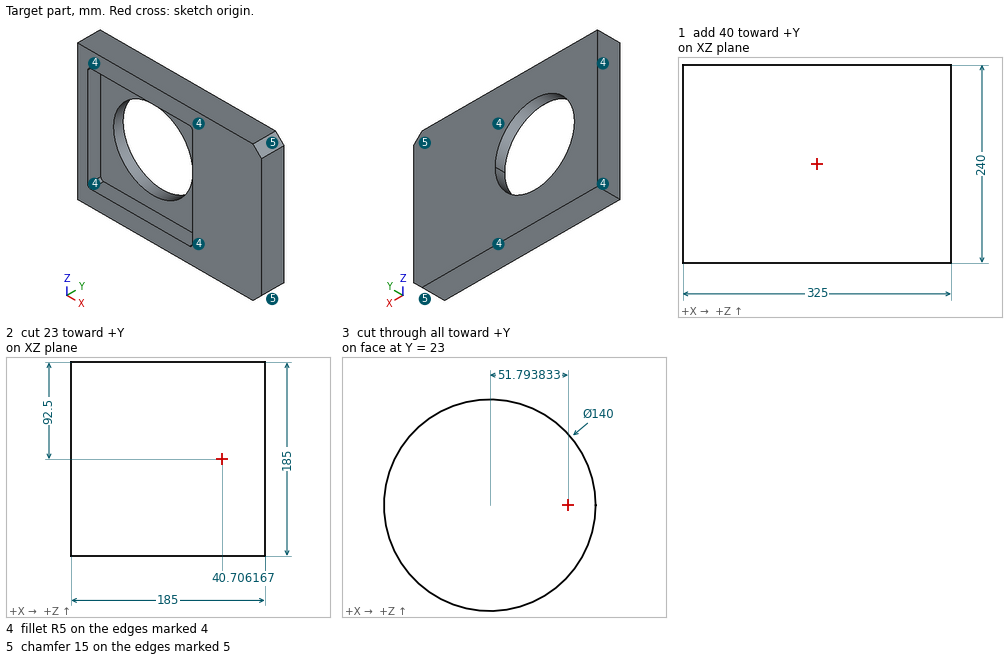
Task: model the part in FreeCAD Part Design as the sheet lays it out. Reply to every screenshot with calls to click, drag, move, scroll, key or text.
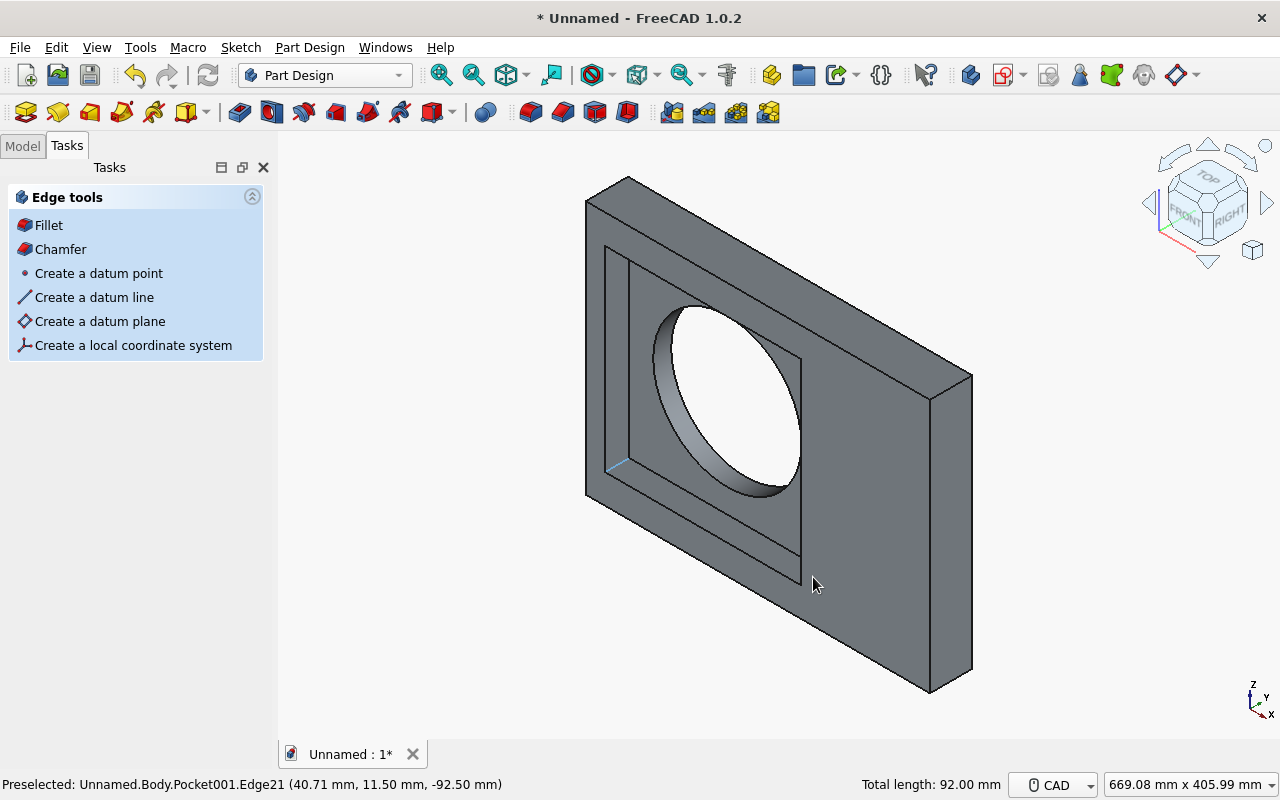
click(532, 112)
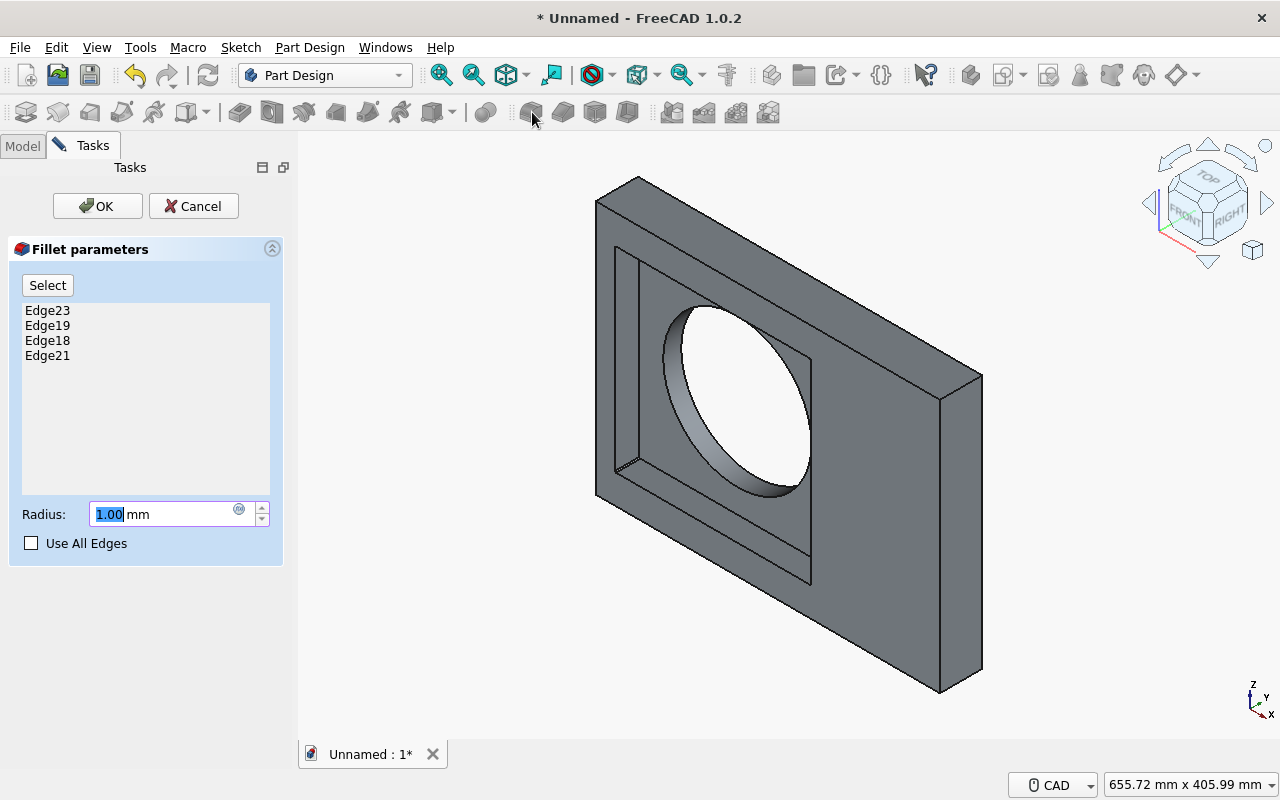
text(5)
key(Tab)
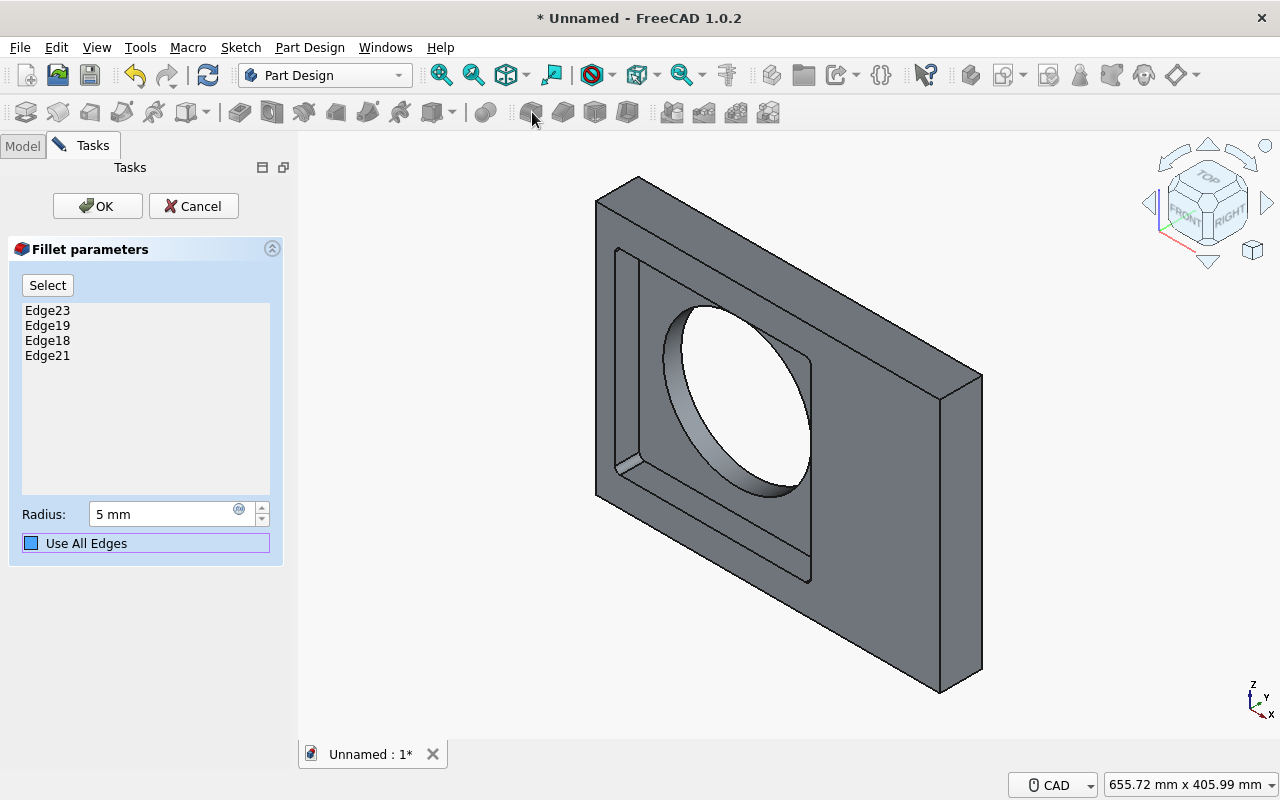
click(98, 206)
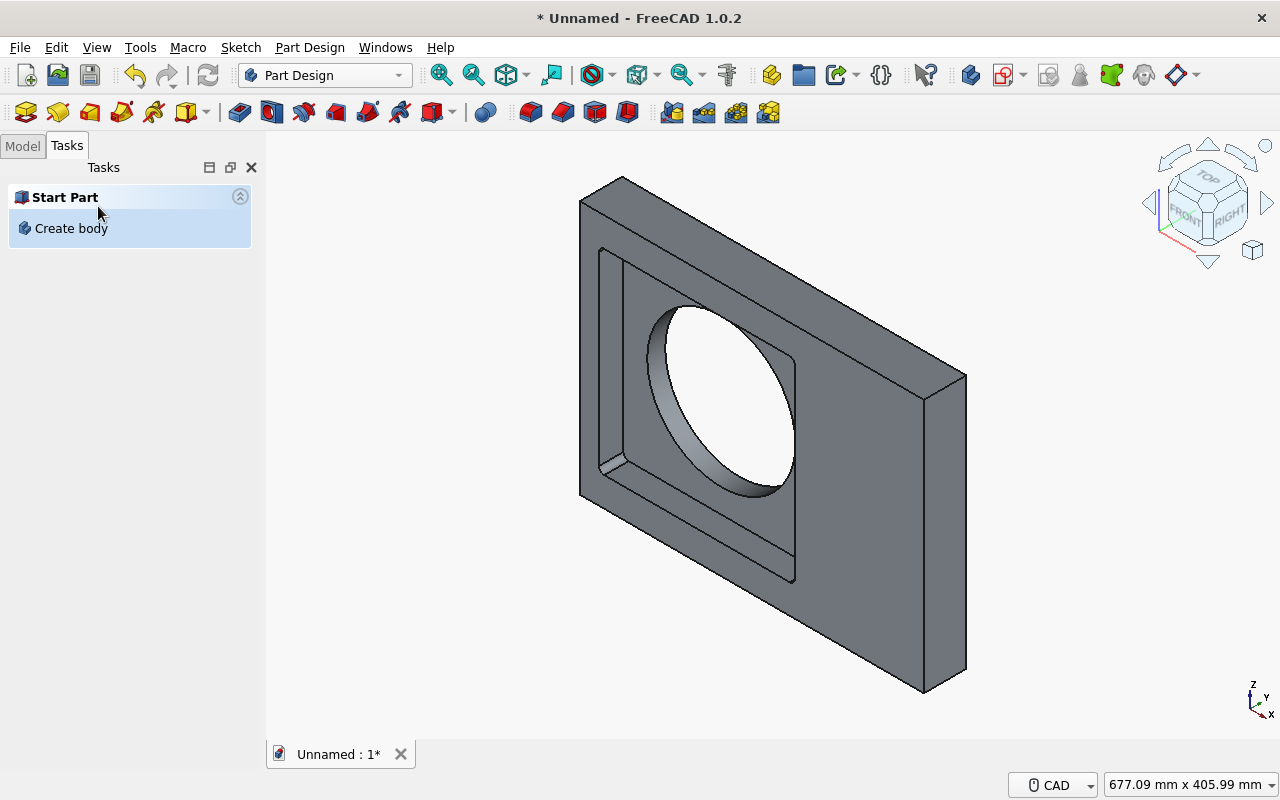
click(945, 387)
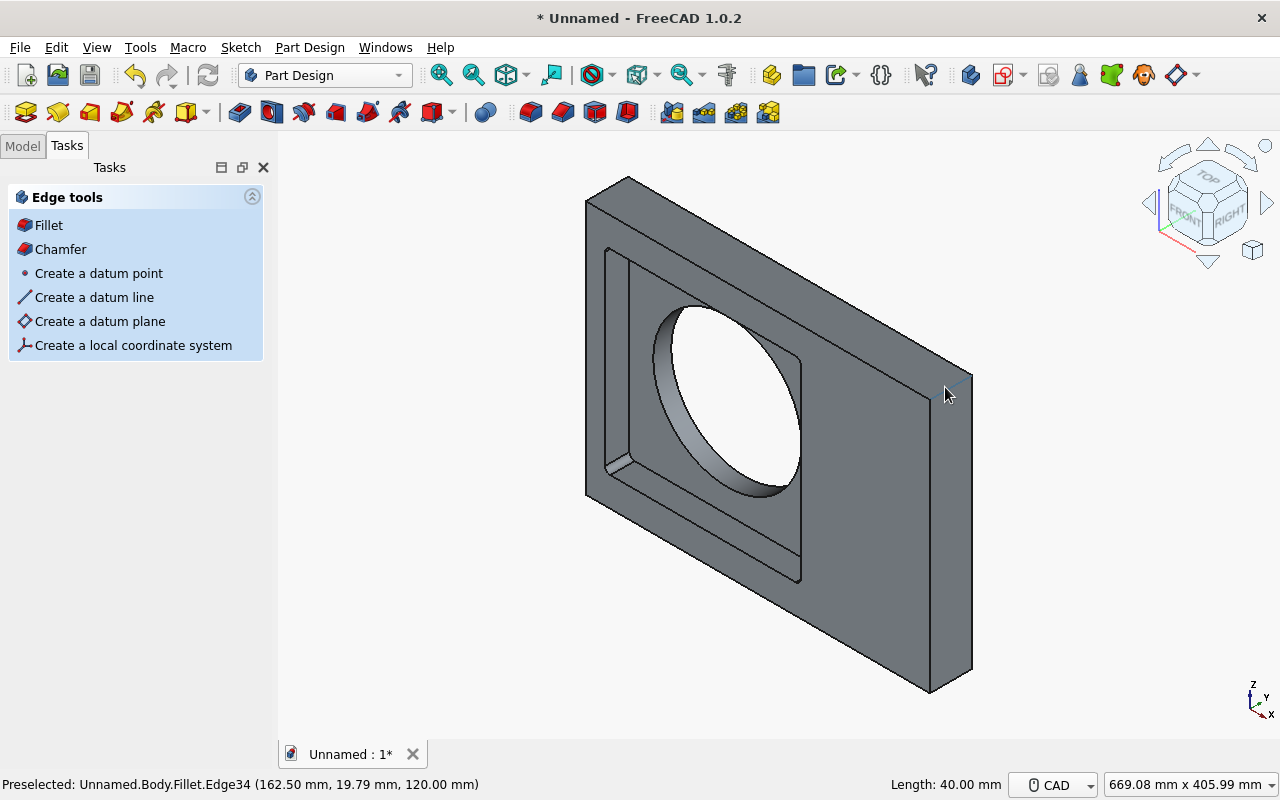
key(2)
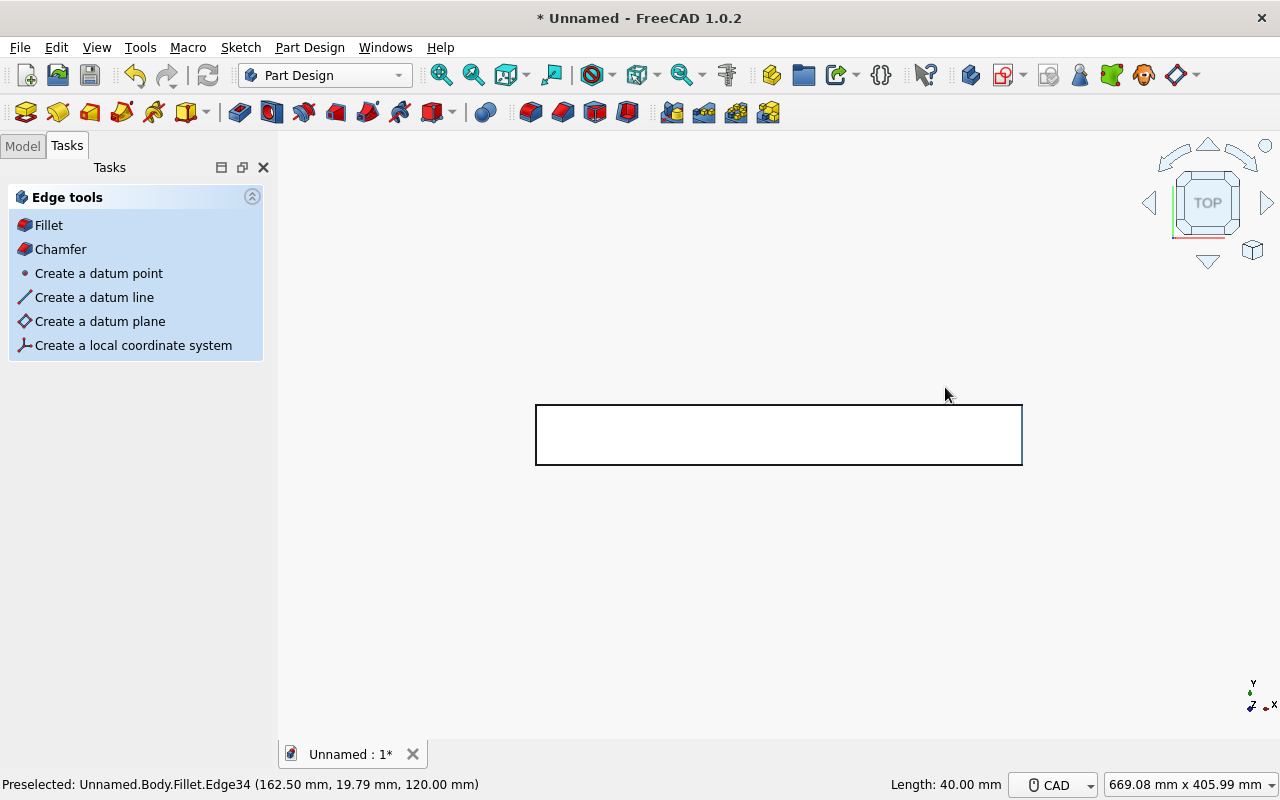
key(0)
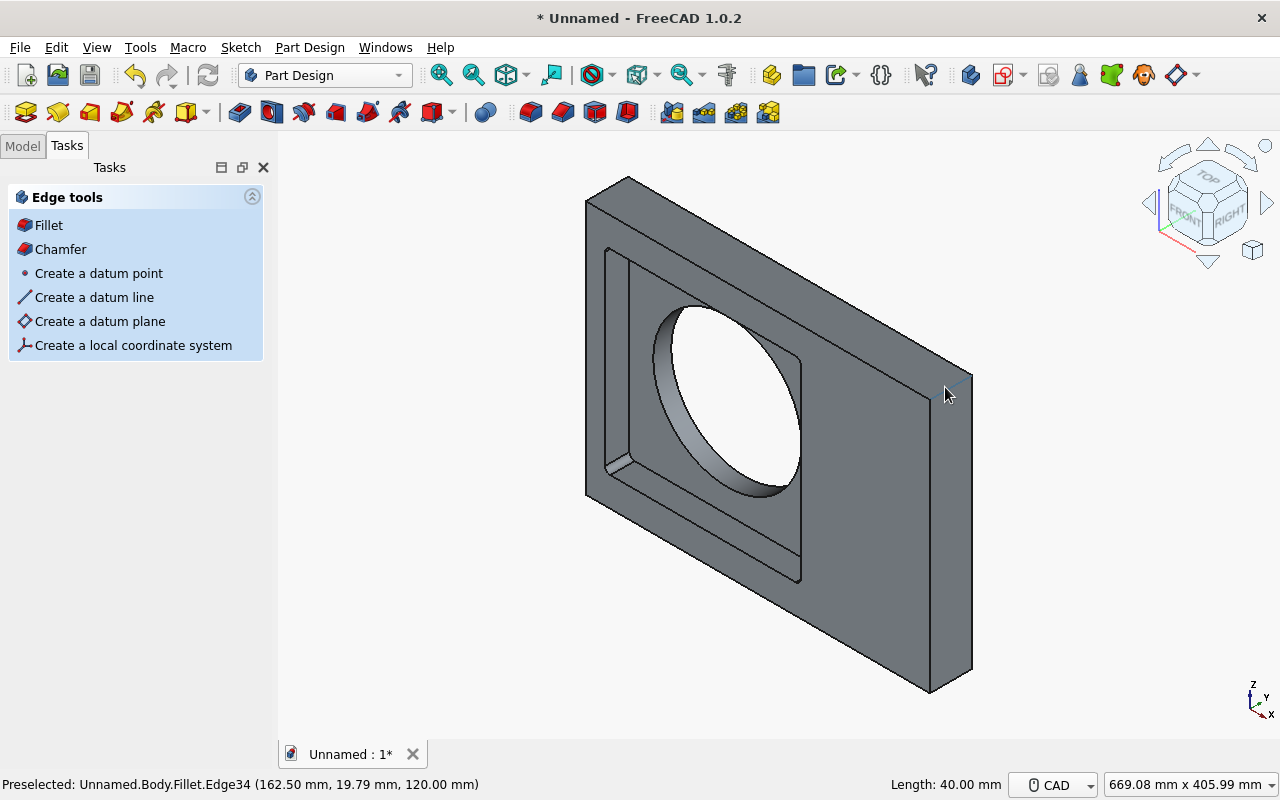
key(1)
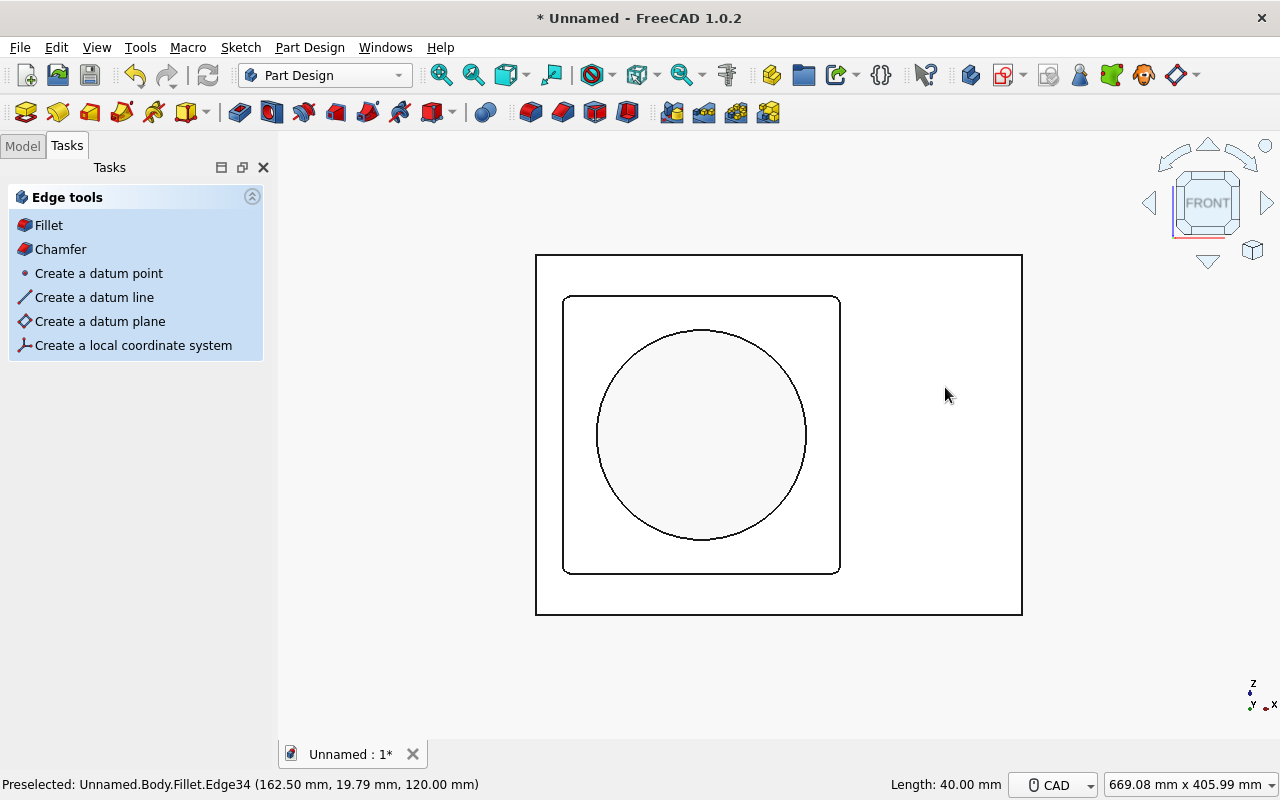
key(3)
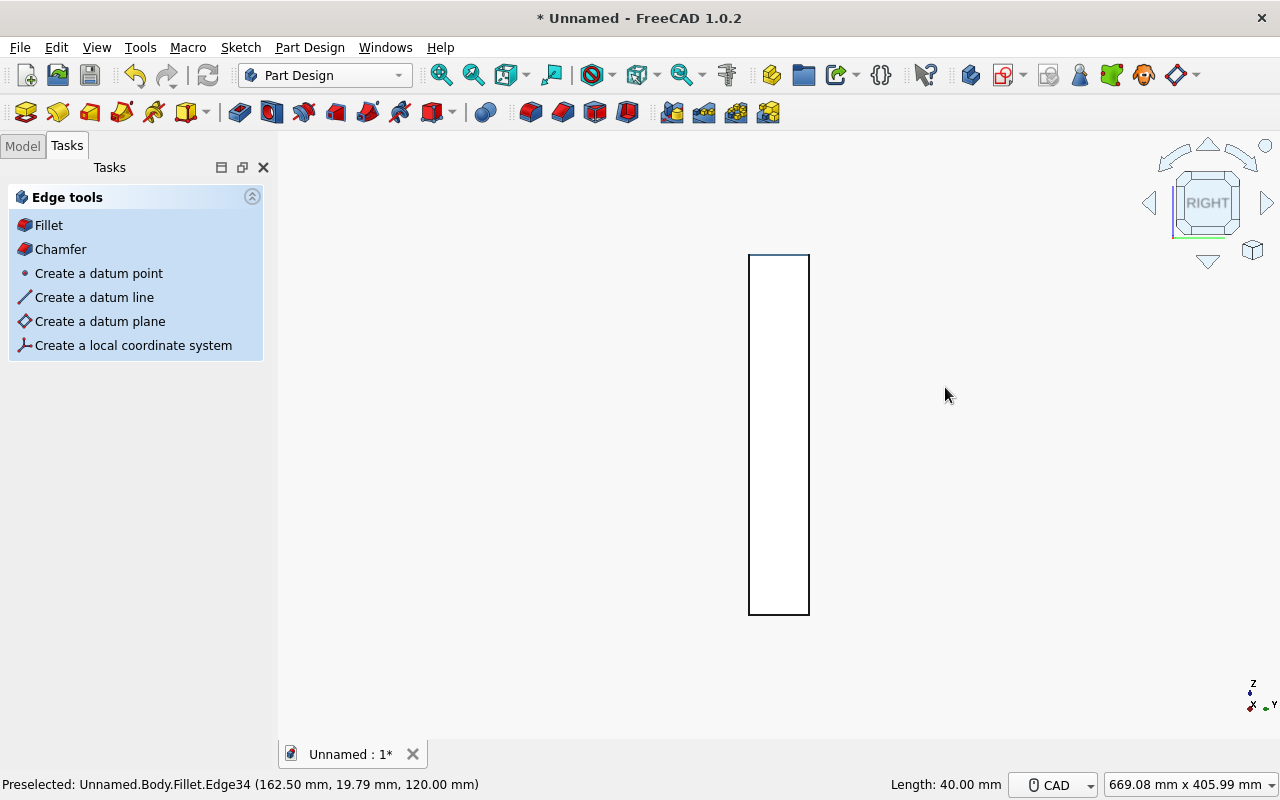
click(779, 614, ctrl)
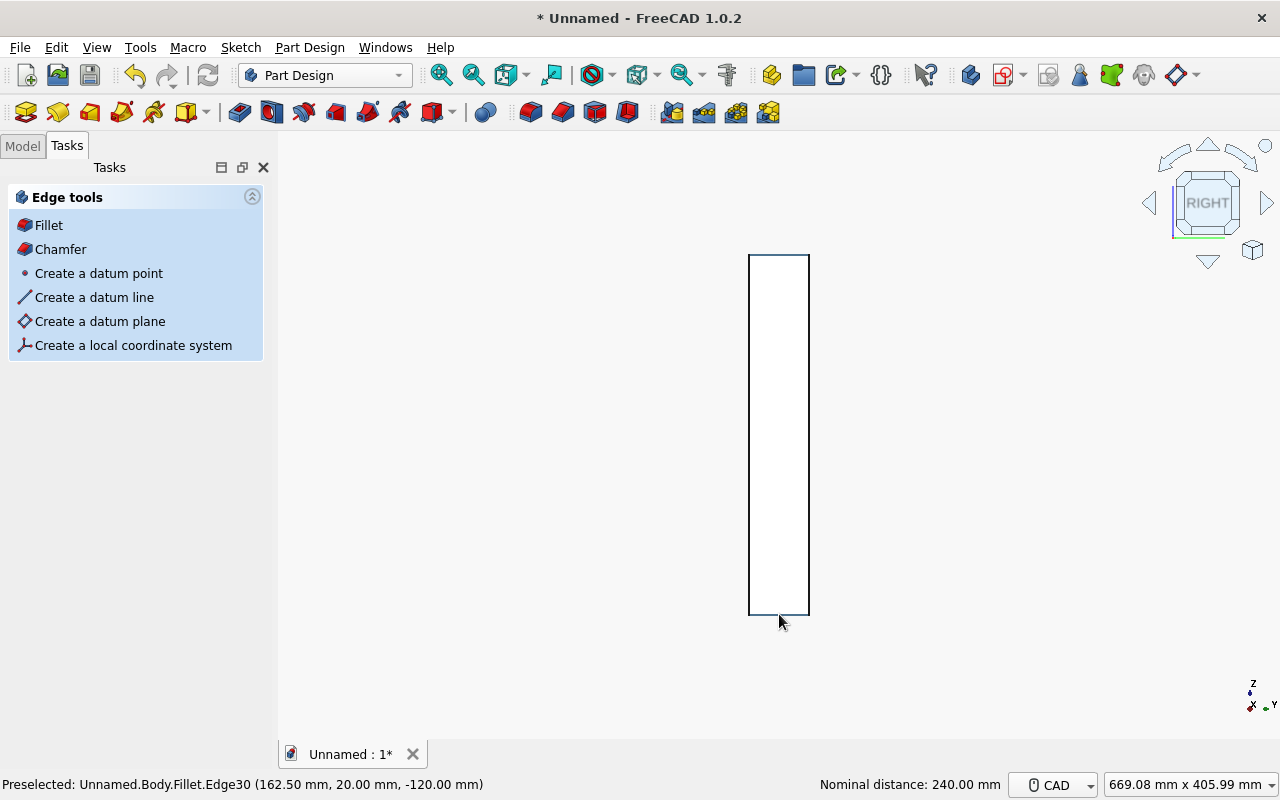
click(564, 112)